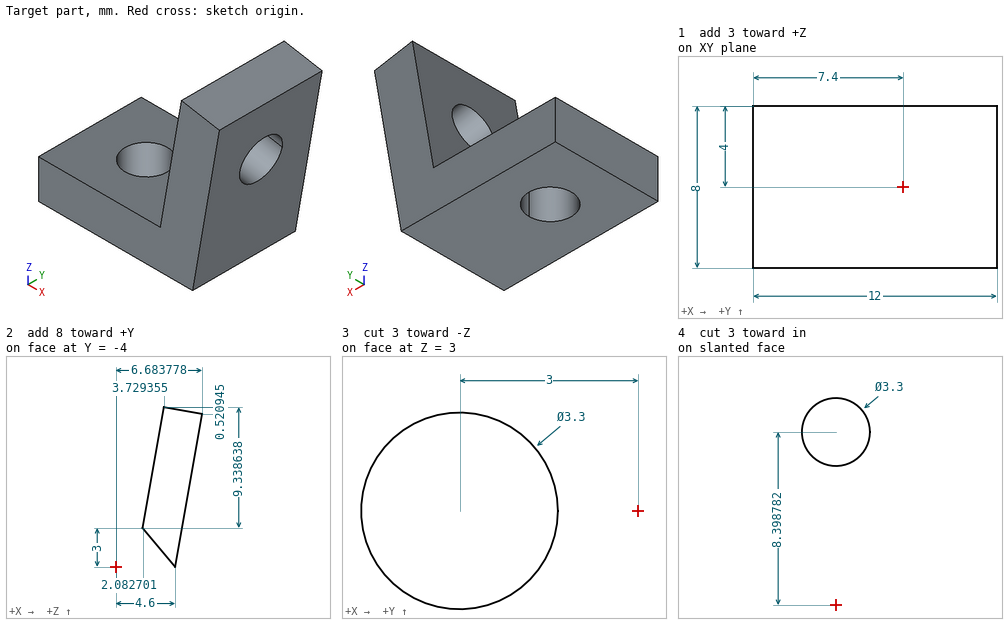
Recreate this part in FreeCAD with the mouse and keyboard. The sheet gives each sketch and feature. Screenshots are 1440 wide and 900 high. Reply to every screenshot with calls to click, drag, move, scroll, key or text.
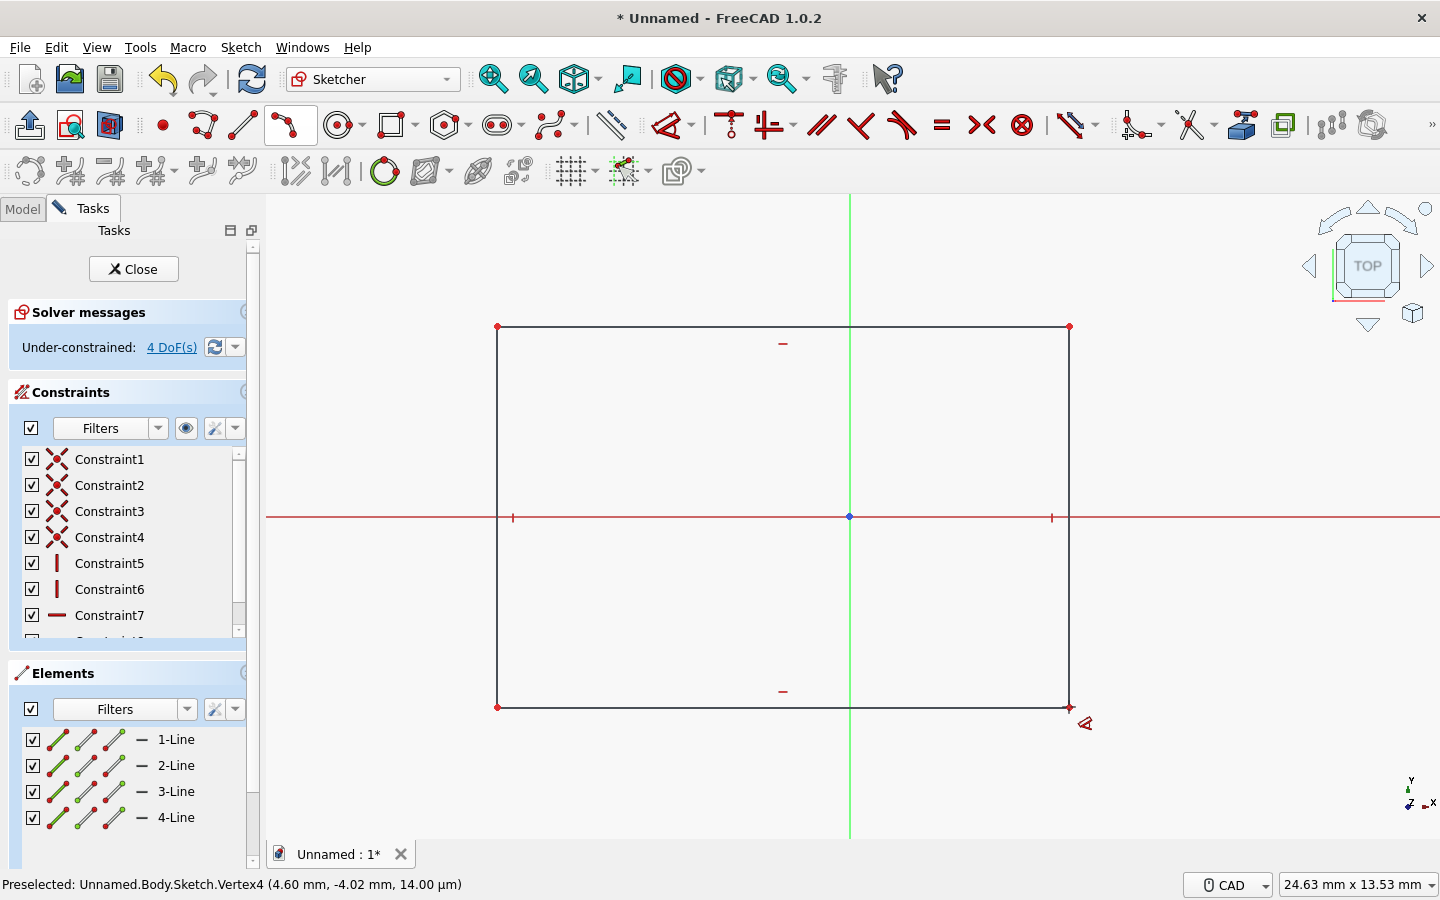
click(497, 441)
click(463, 430)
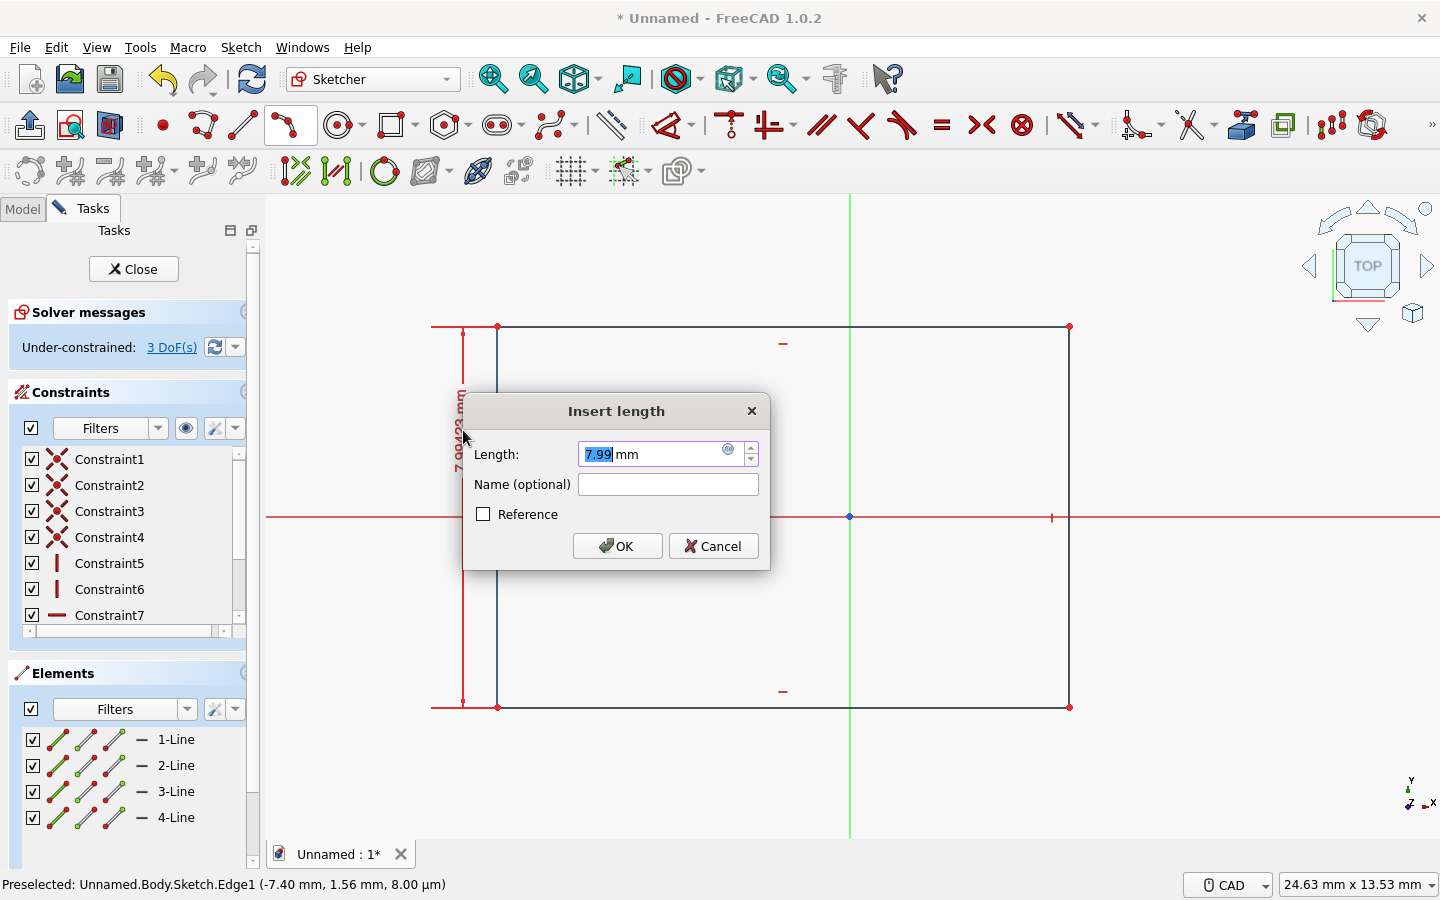
text(8)
key(Return)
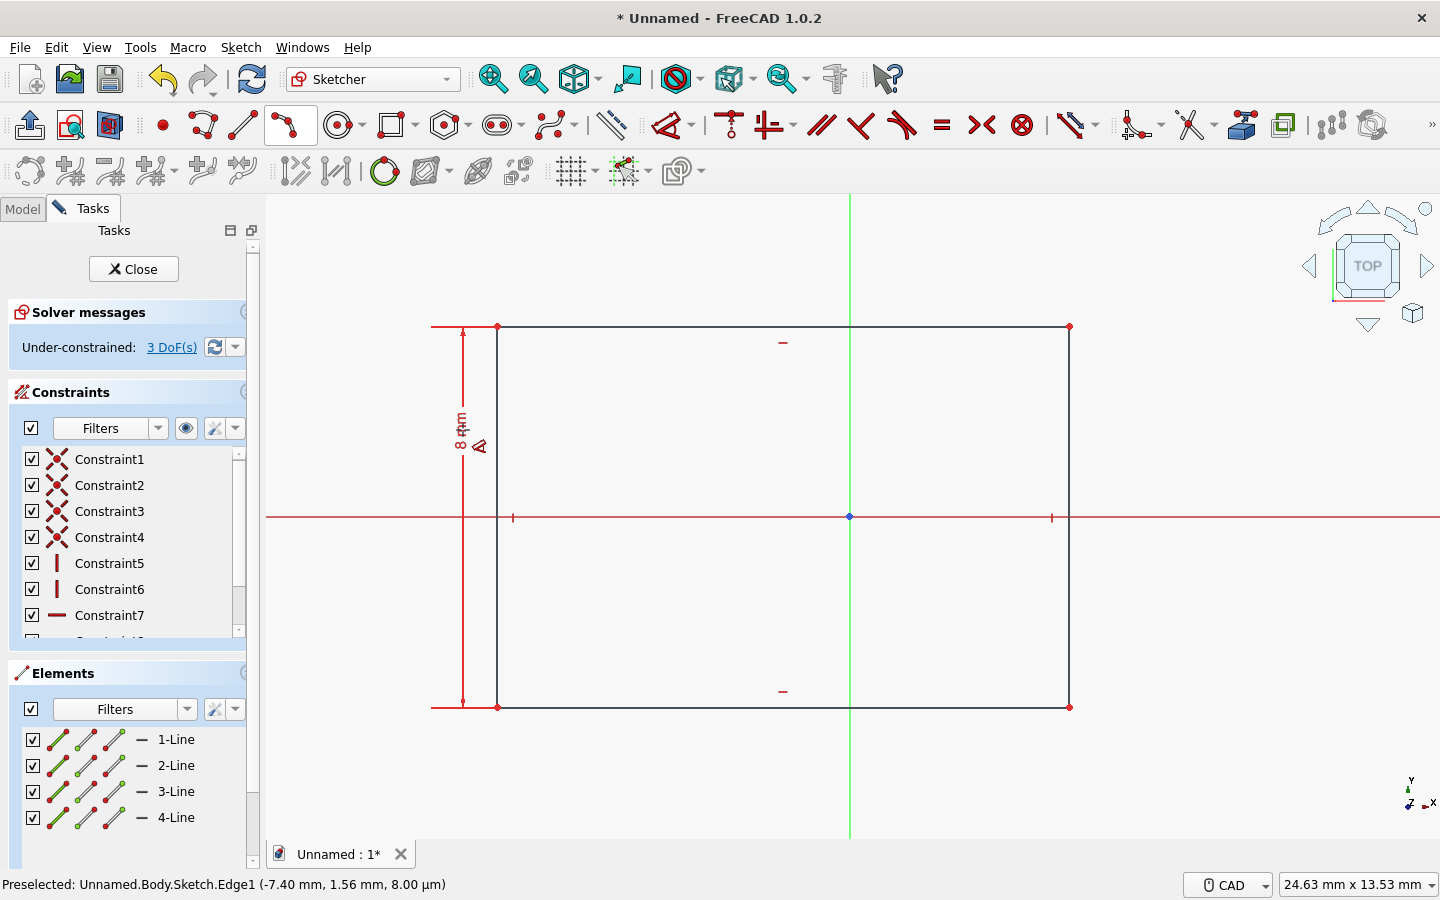
click(669, 708)
click(783, 742)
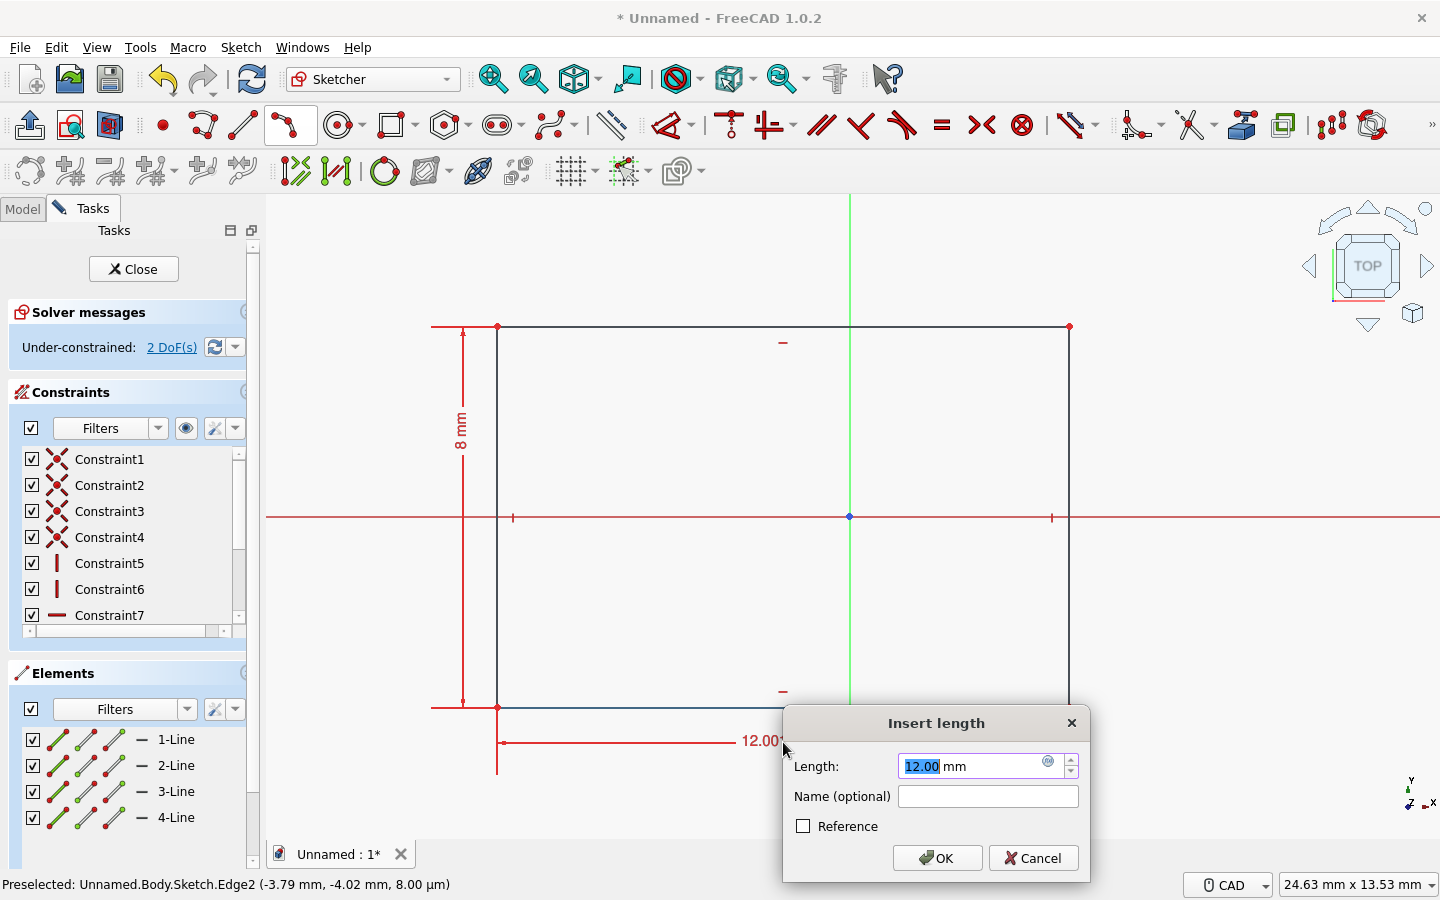
text(12)
key(Return)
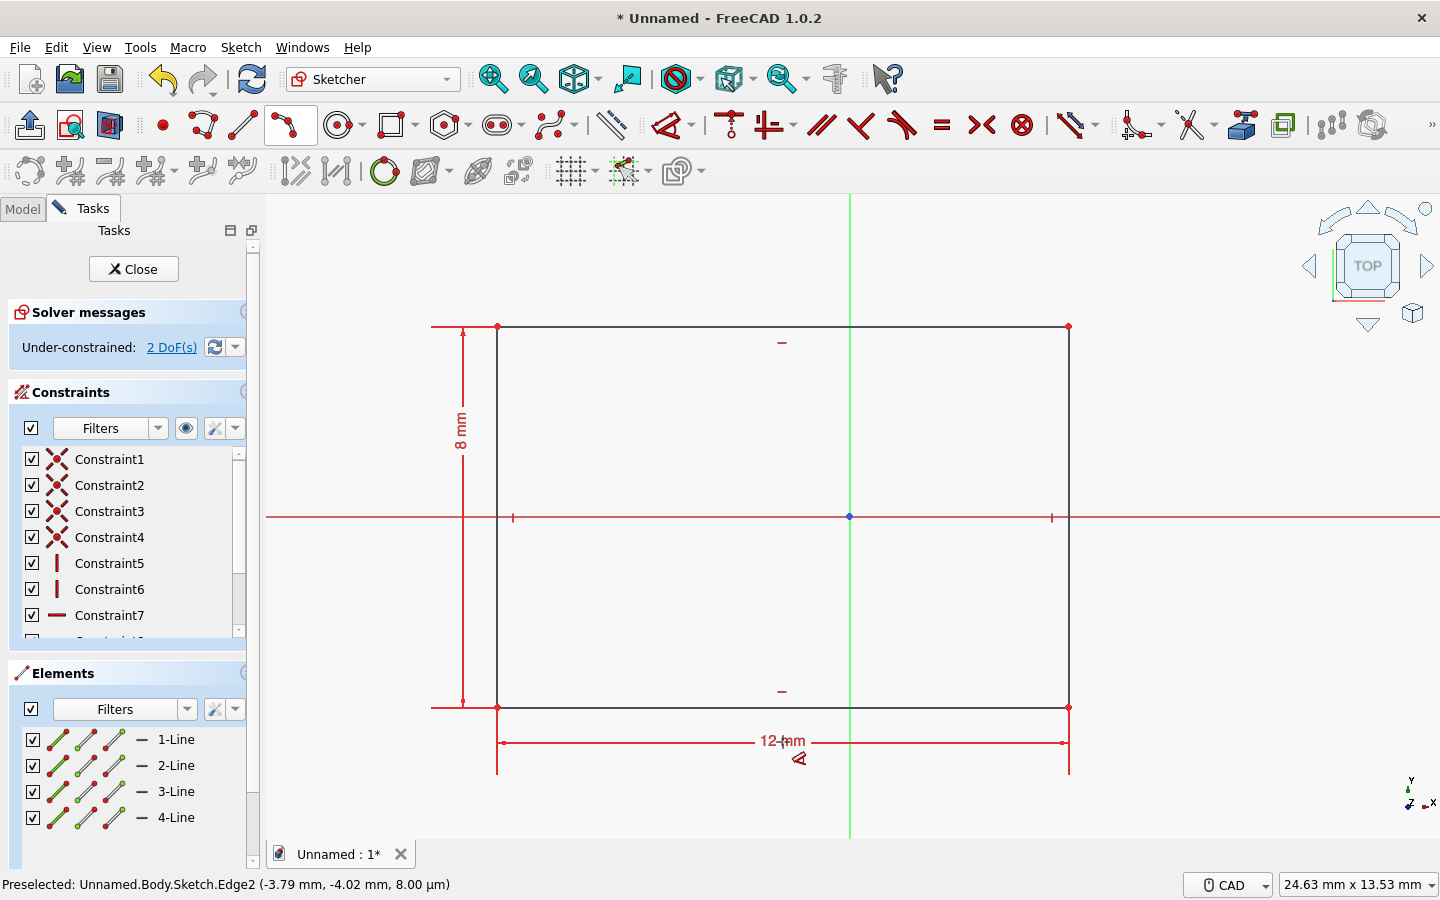
click(497, 327)
click(463, 378)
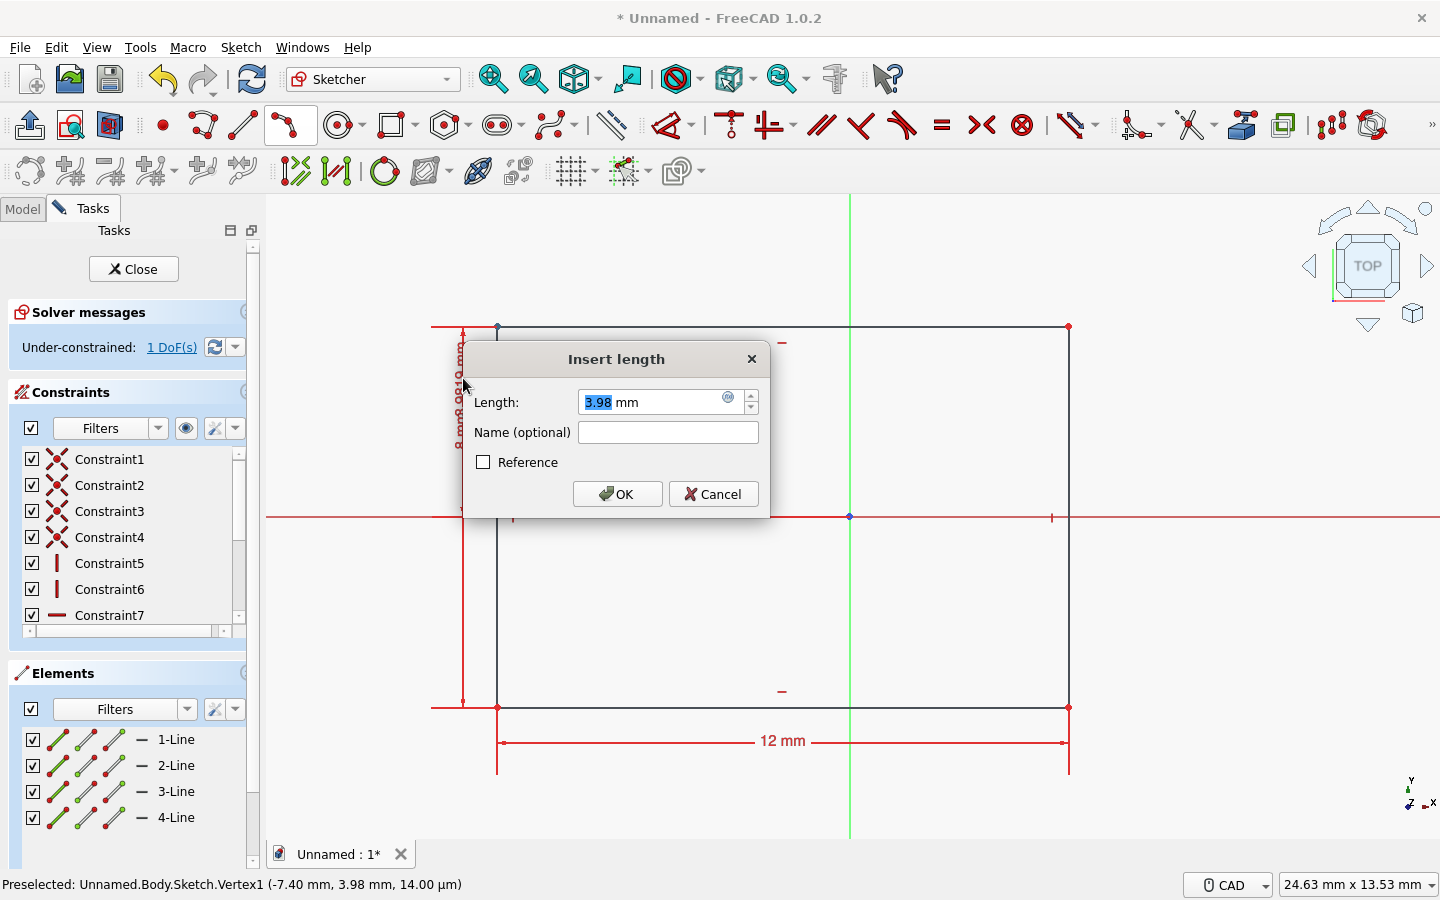
text(4)
key(Return)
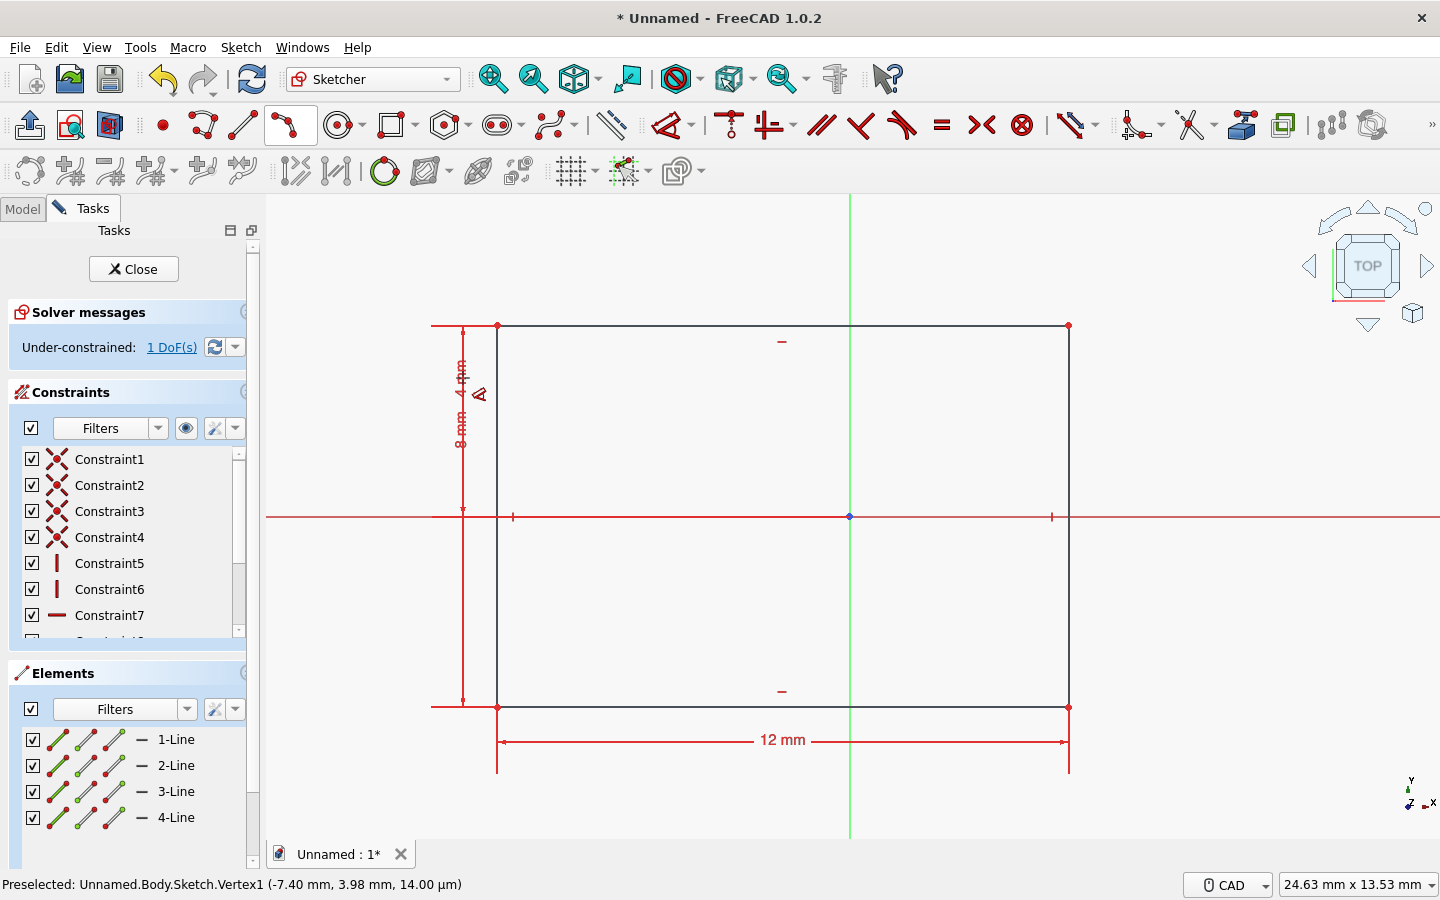
click(497, 326)
click(673, 292)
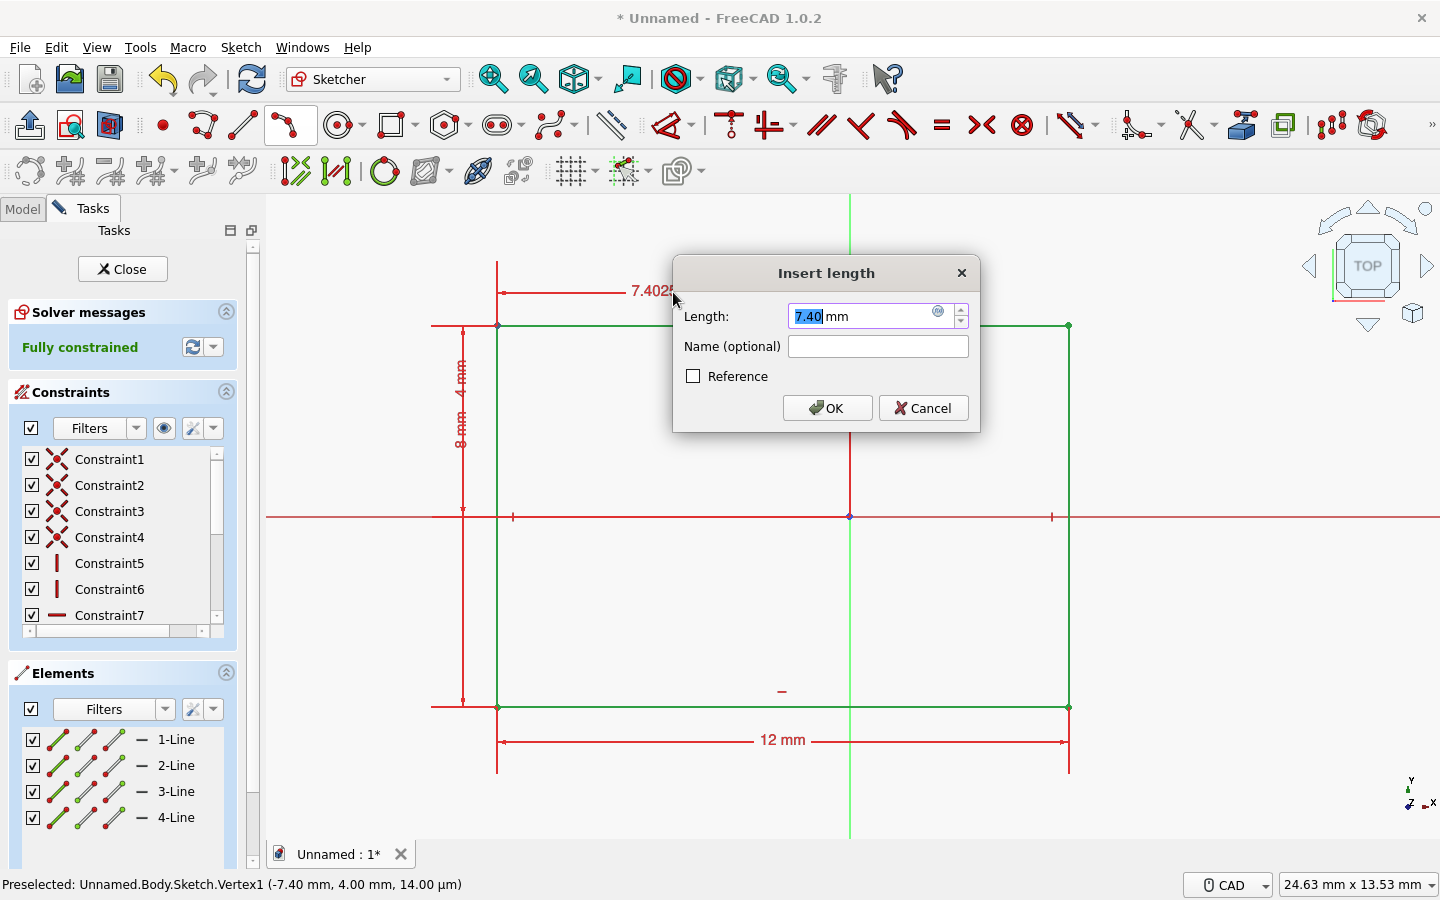
text(7.4)
key(Return)
key(Escape)